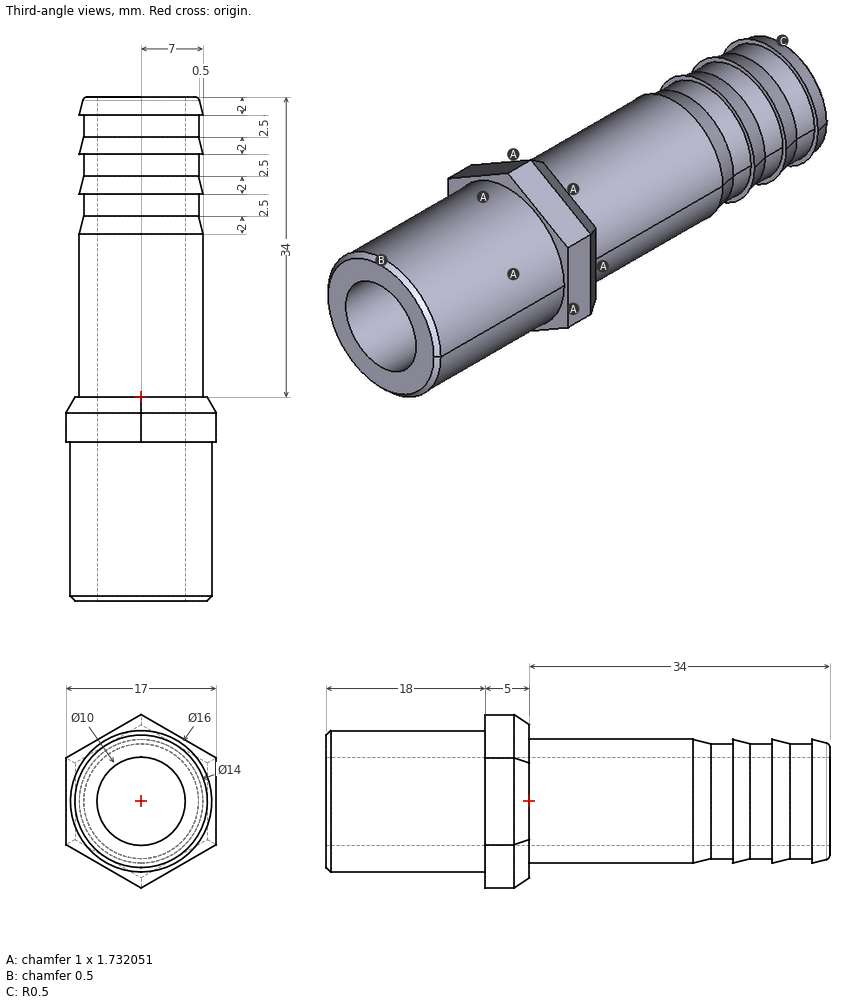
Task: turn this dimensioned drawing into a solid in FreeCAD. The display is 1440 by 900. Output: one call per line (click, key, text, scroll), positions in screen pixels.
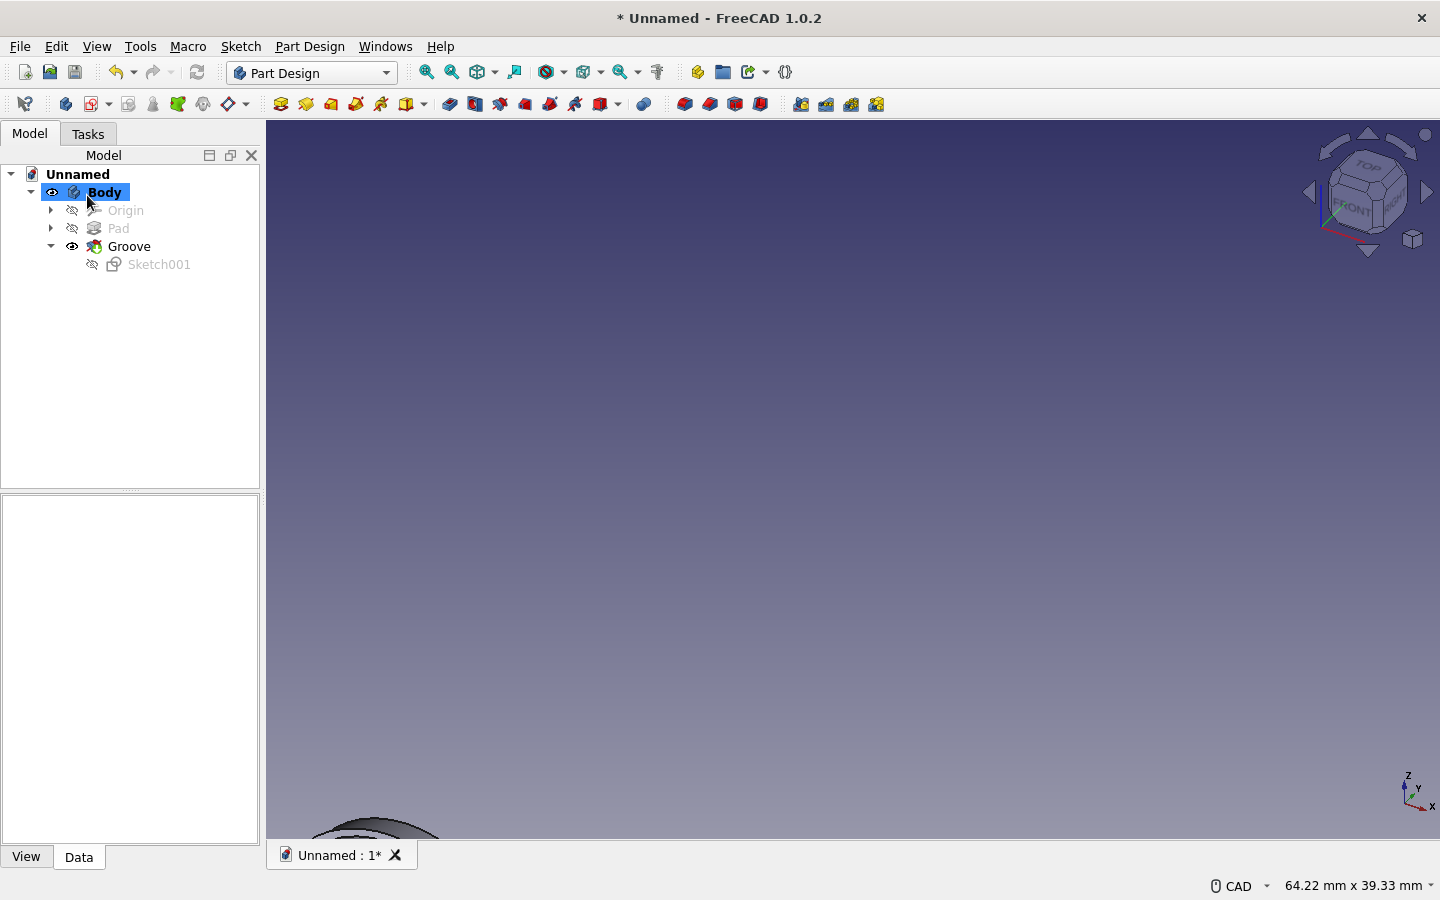
click(427, 72)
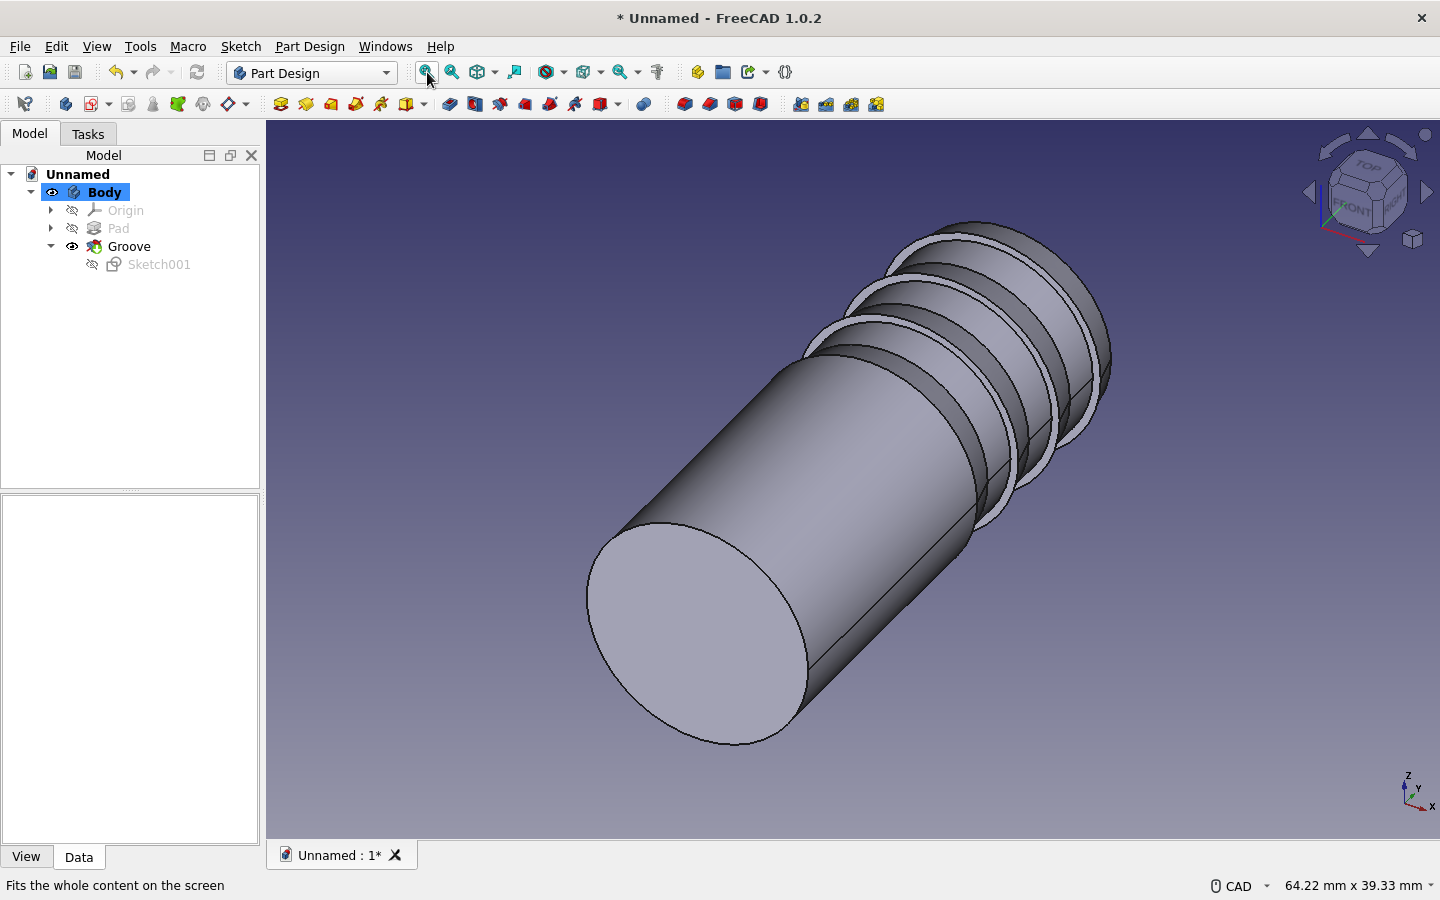
click(697, 633)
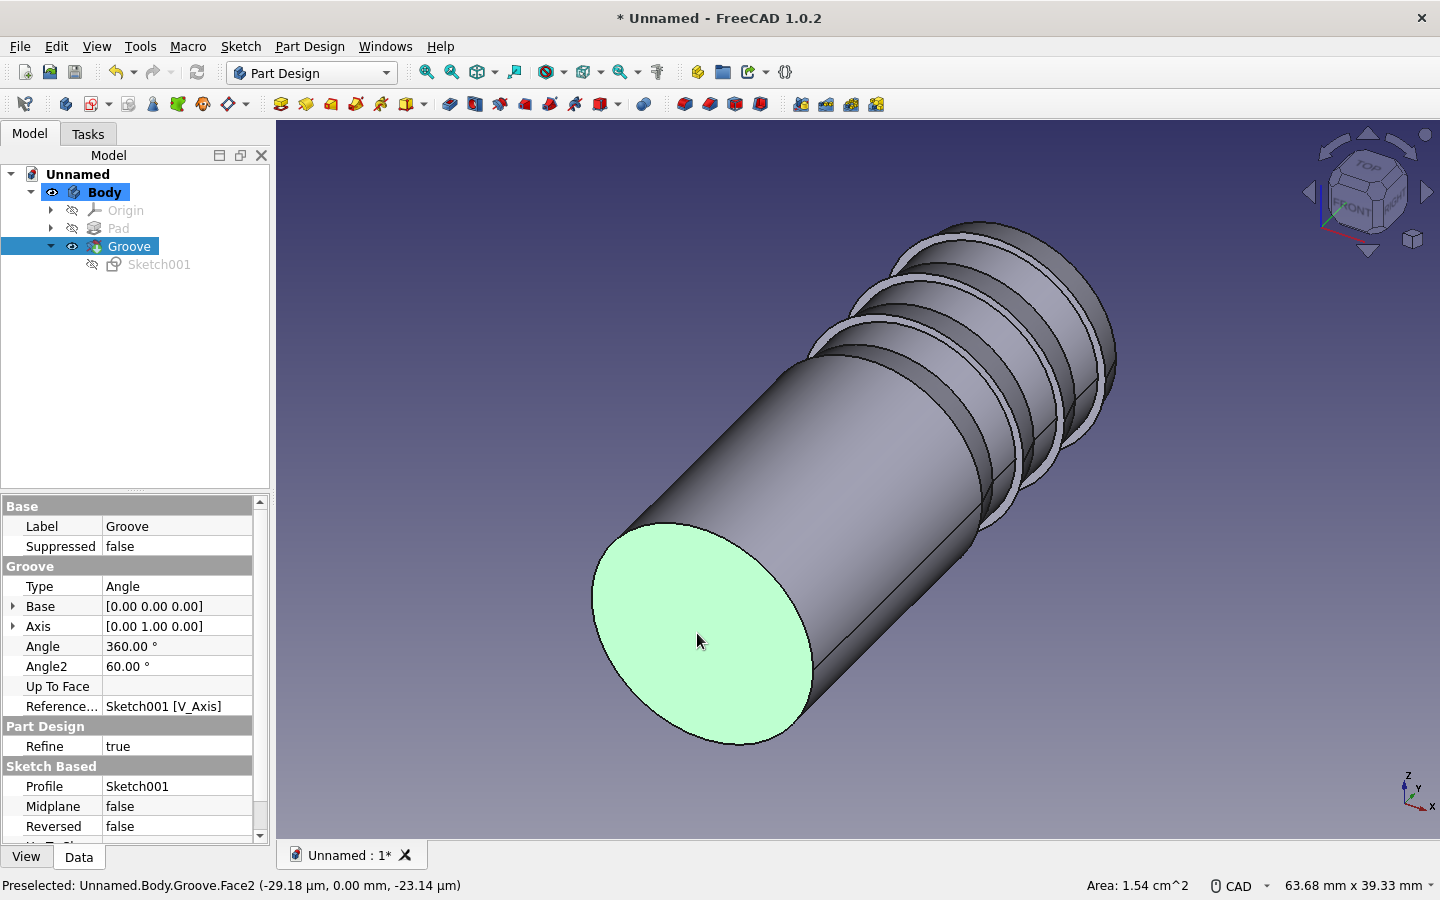
click(90, 104)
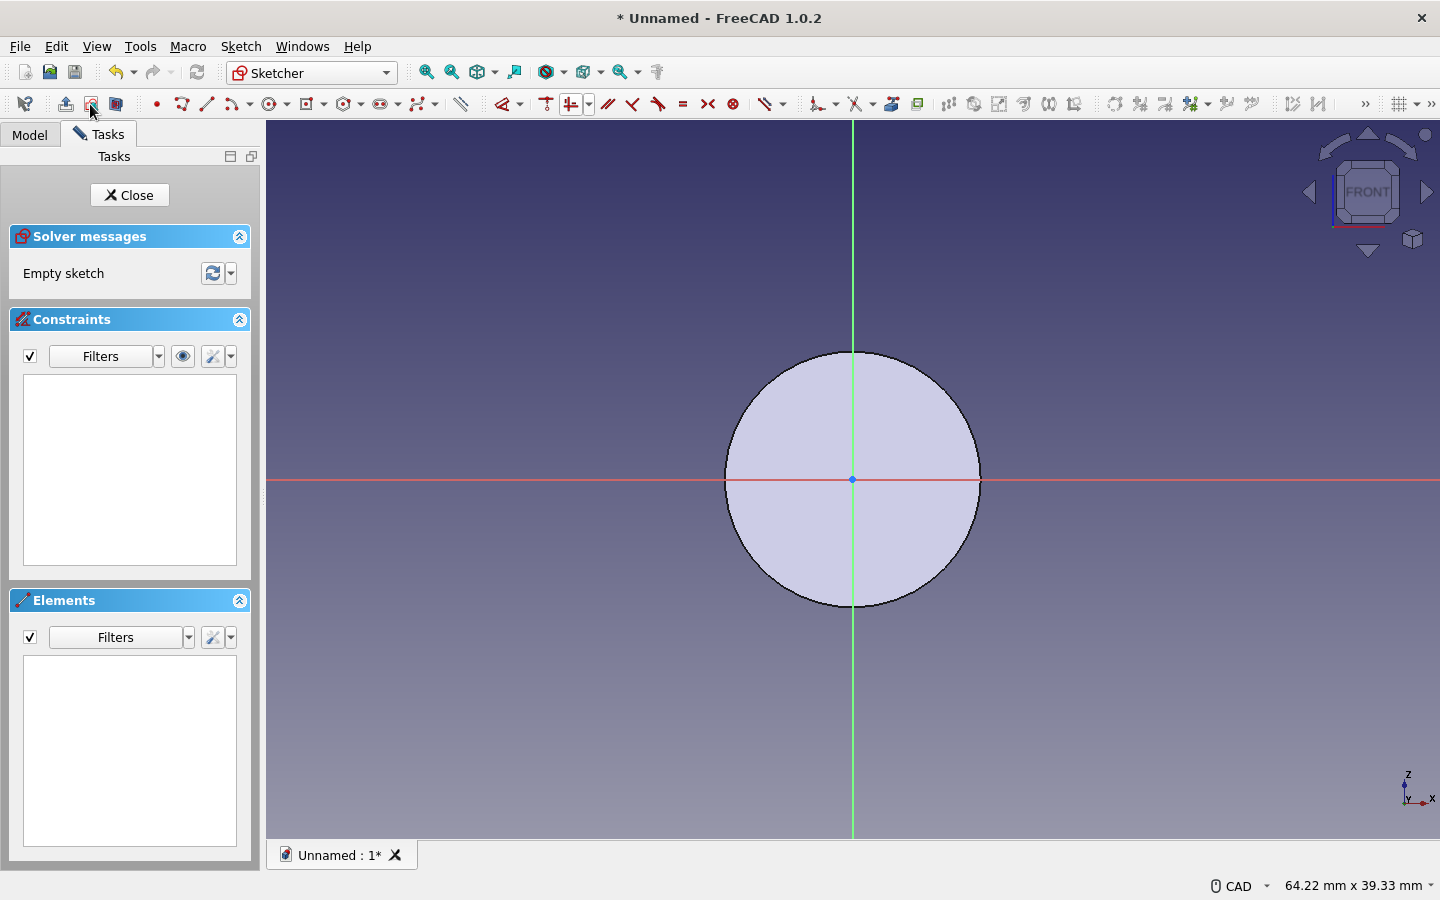
key(g)
key(p)
key(6)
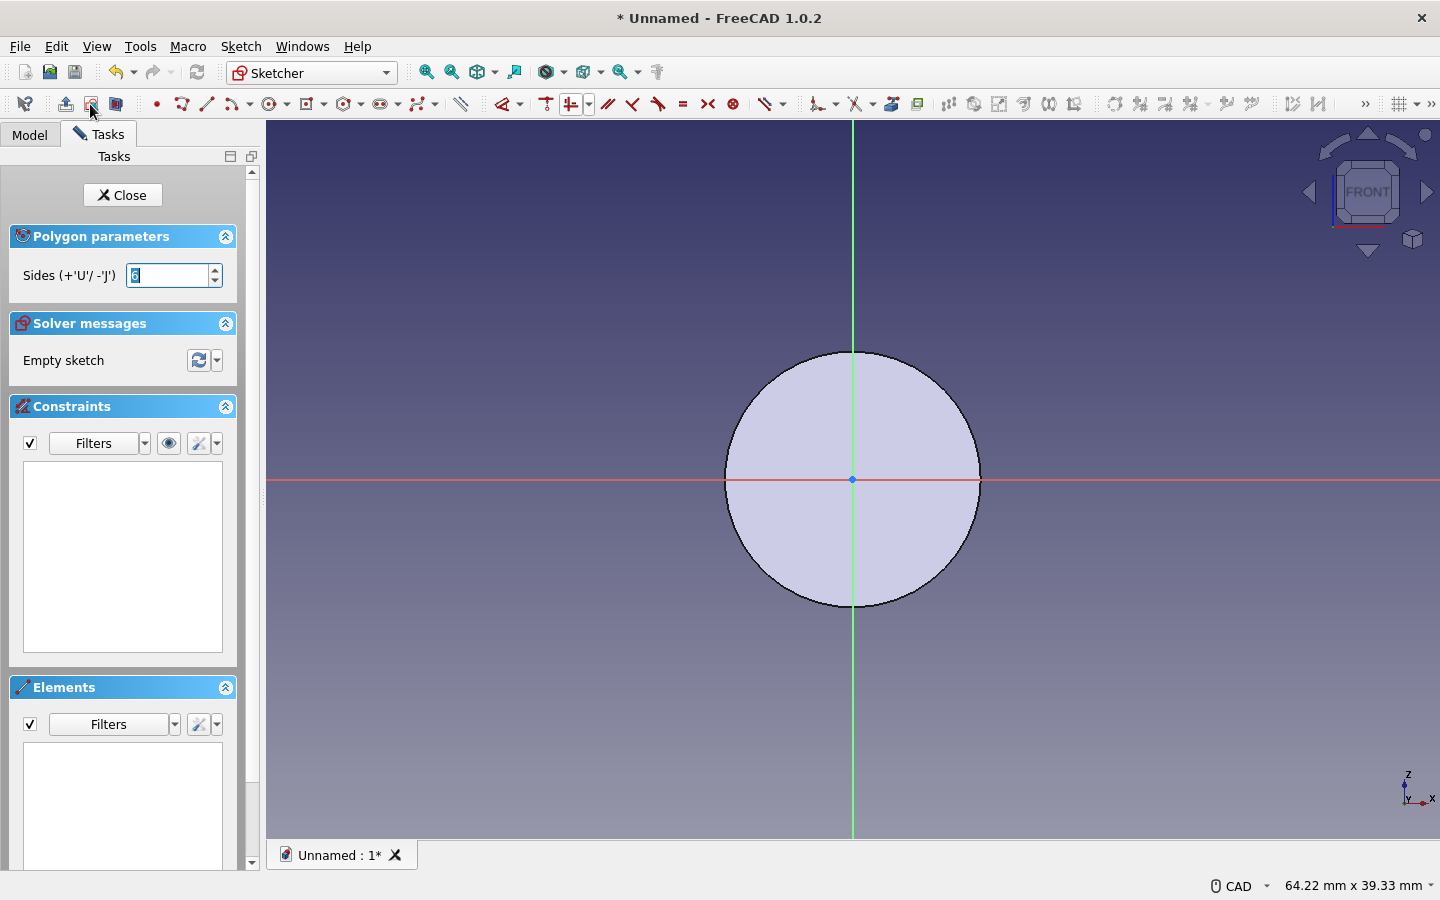
click(853, 480)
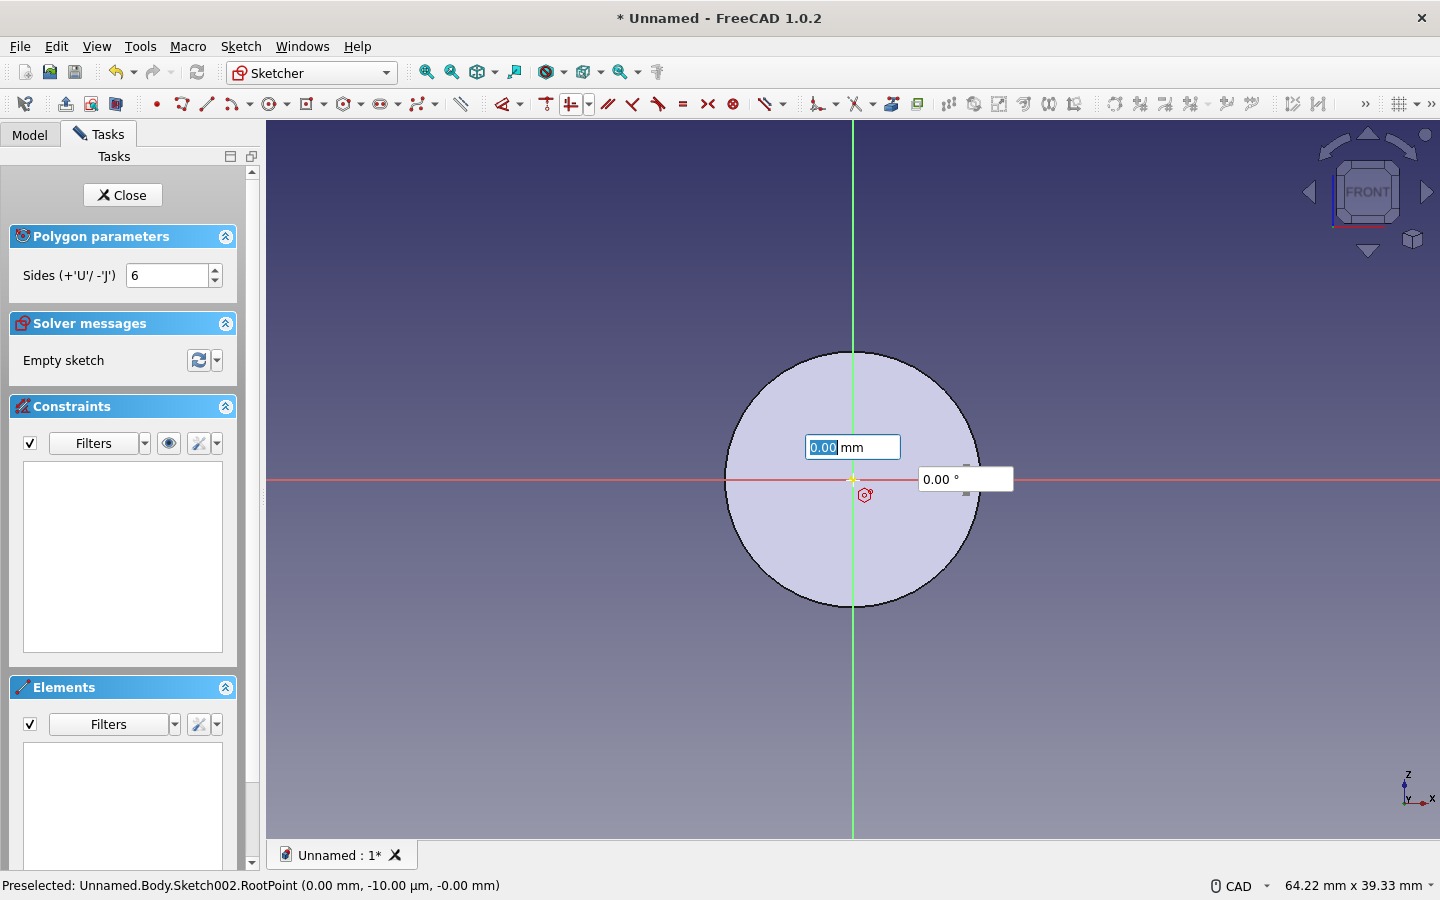
click(853, 300)
key(Escape)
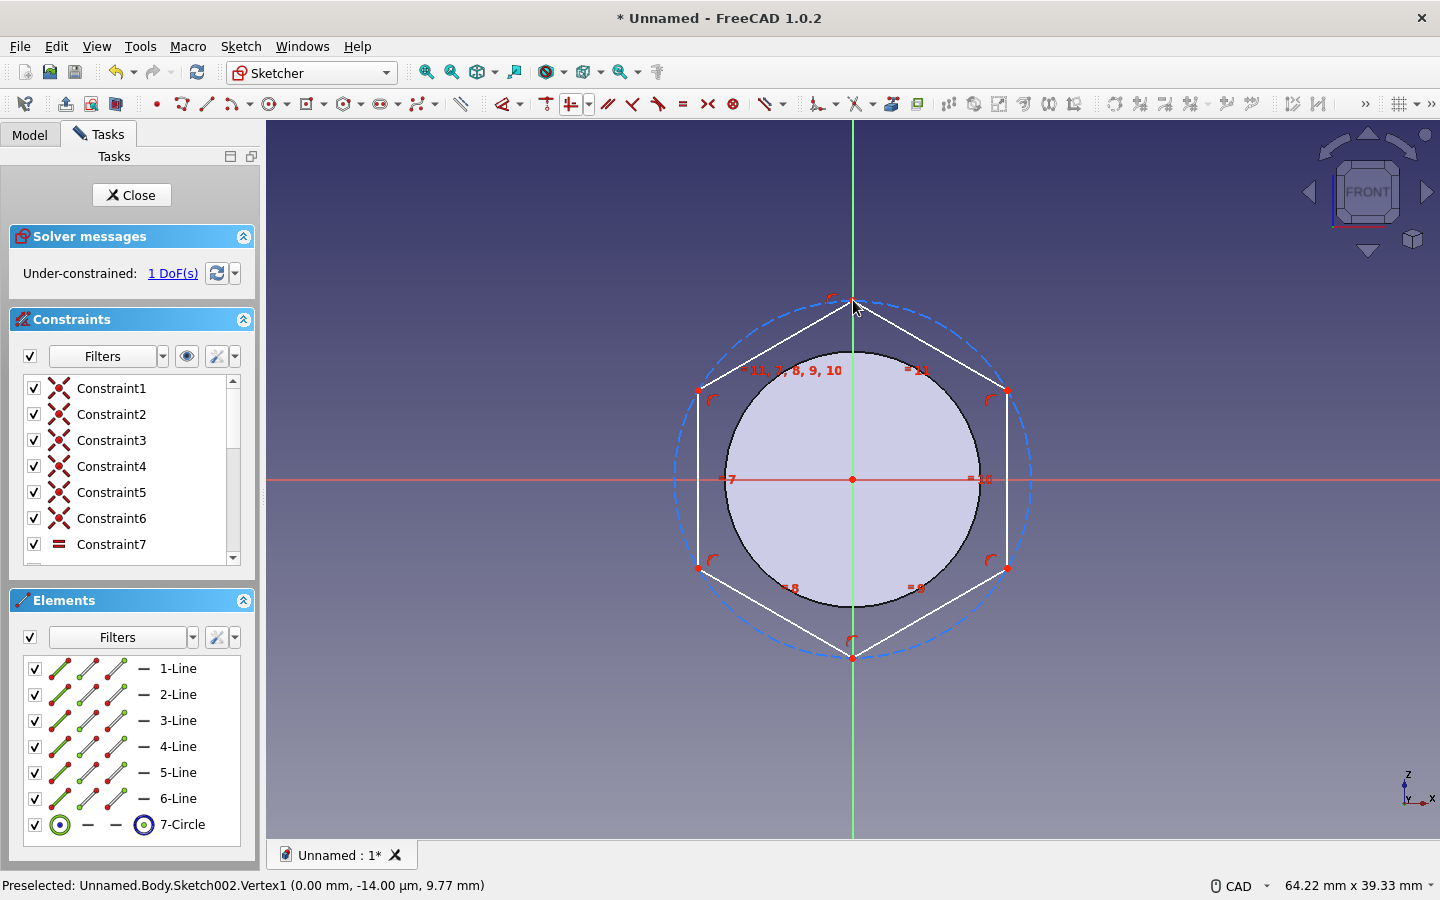
click(502, 104)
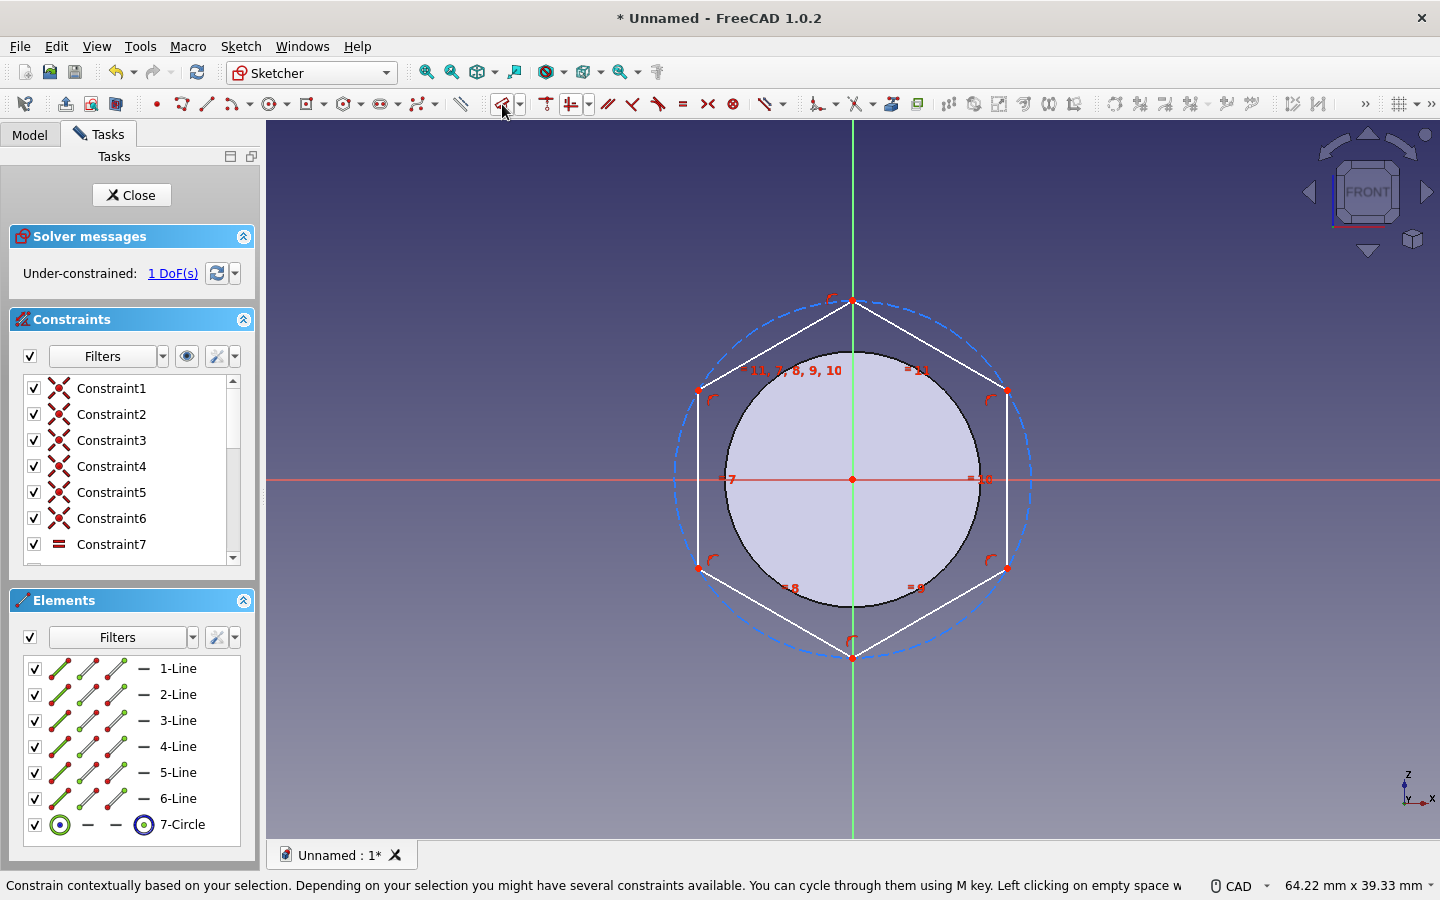
click(698, 390)